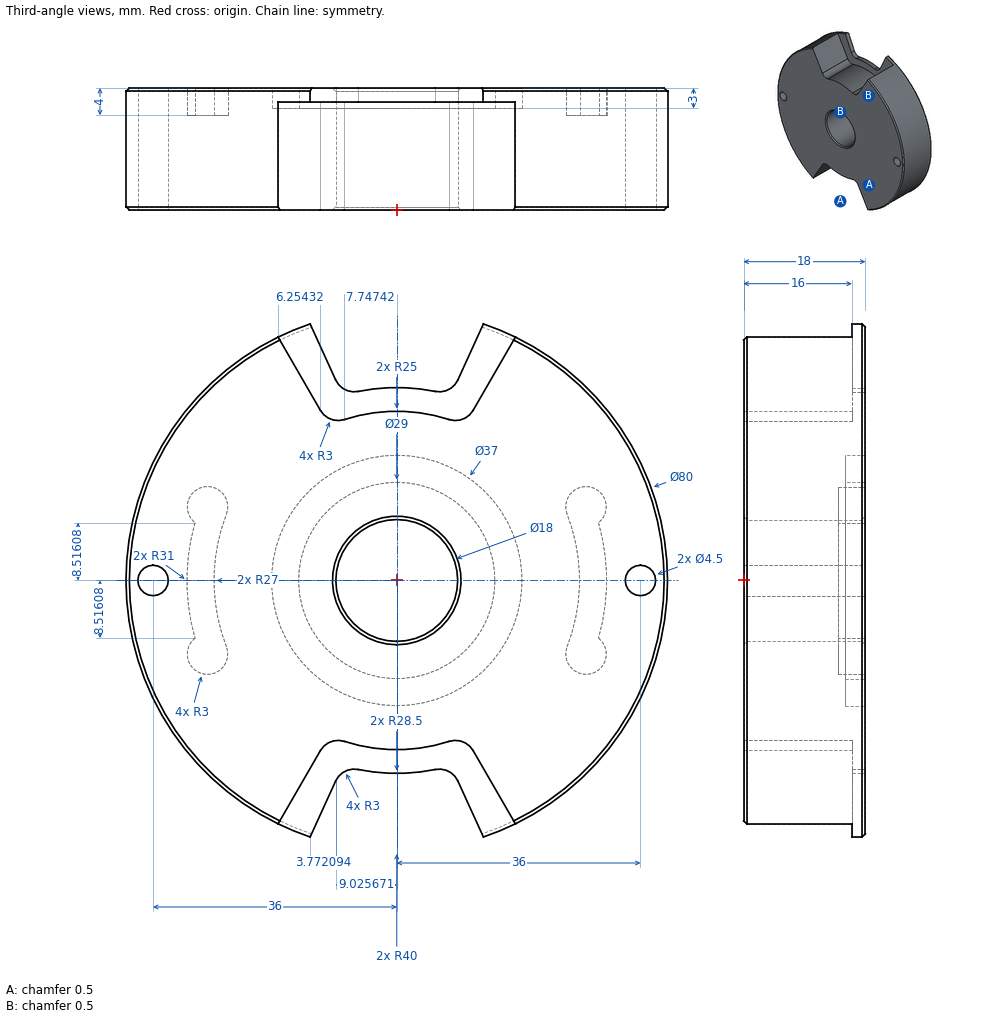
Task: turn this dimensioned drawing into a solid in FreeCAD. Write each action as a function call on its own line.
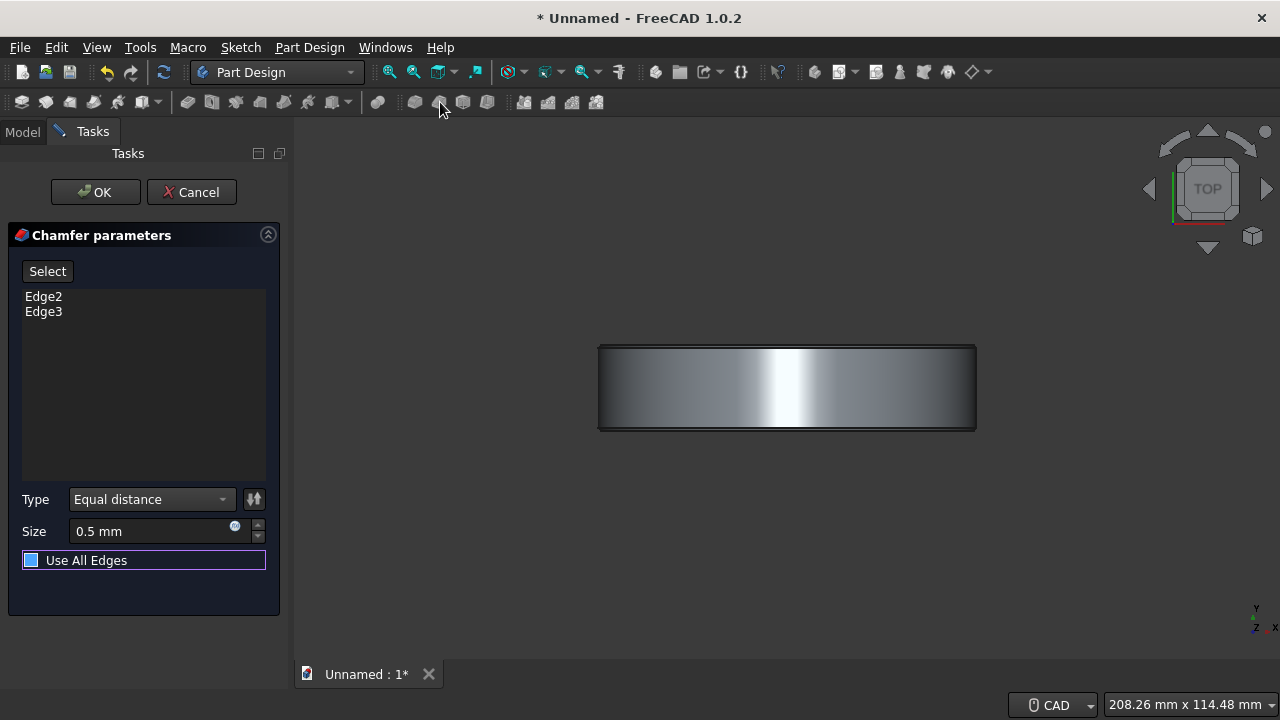
click(96, 192)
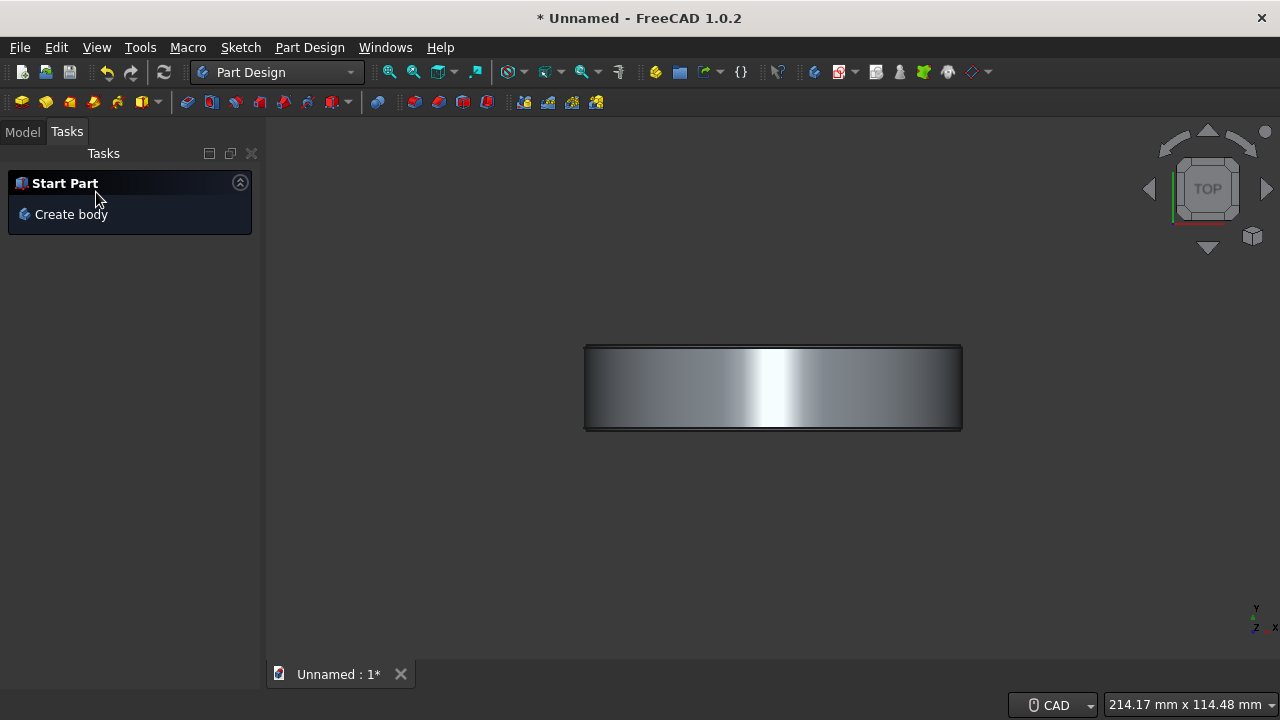
click(390, 72)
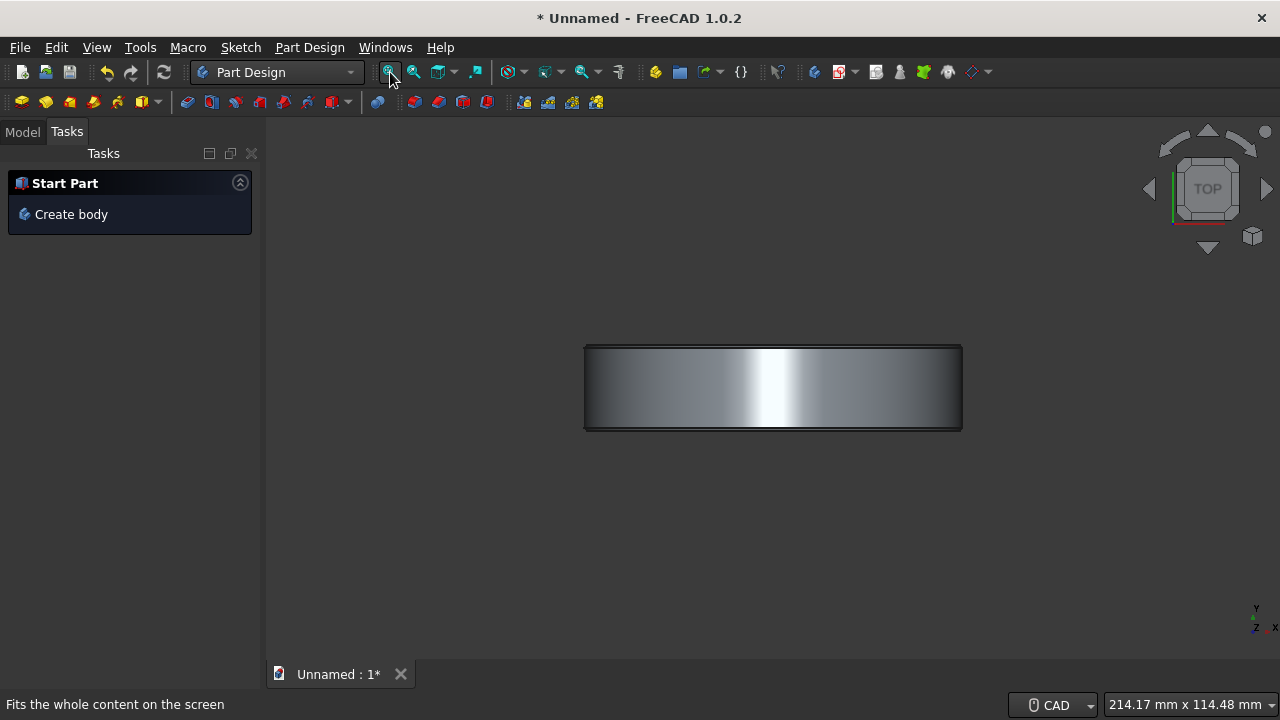
key(4)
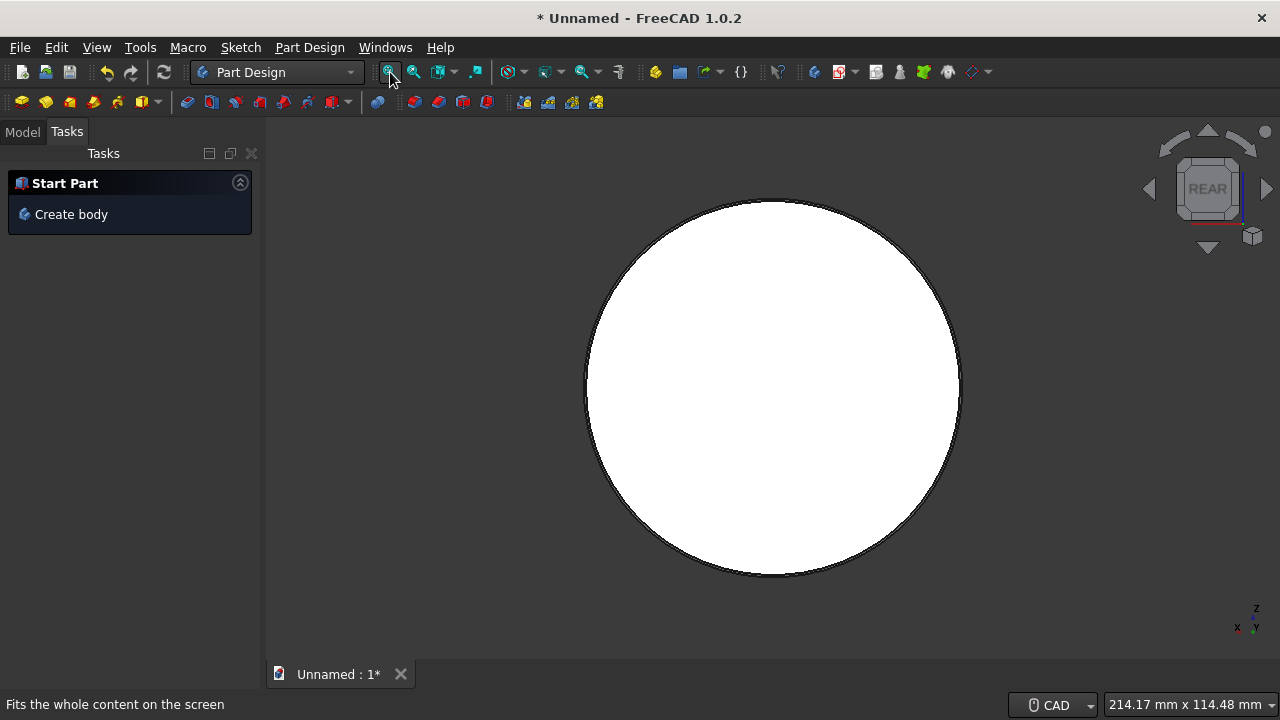
click(773, 387)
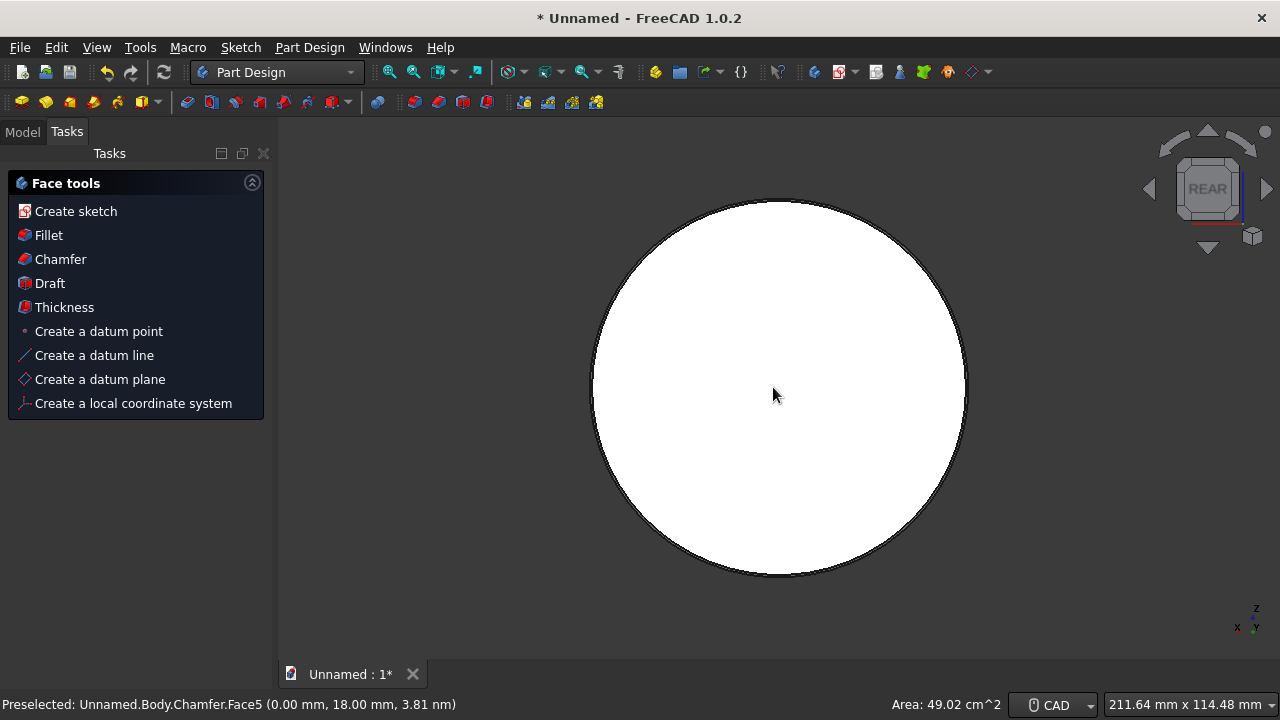
click(840, 72)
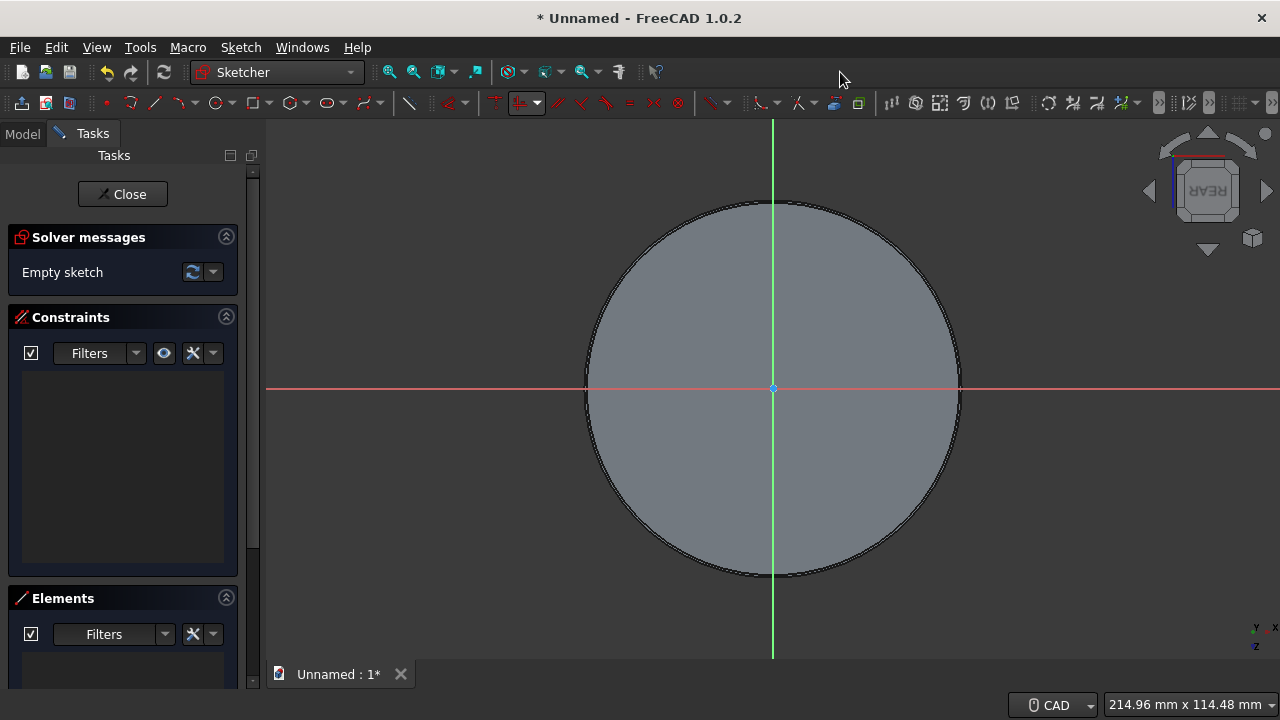
scroll(912, 389, up, 2)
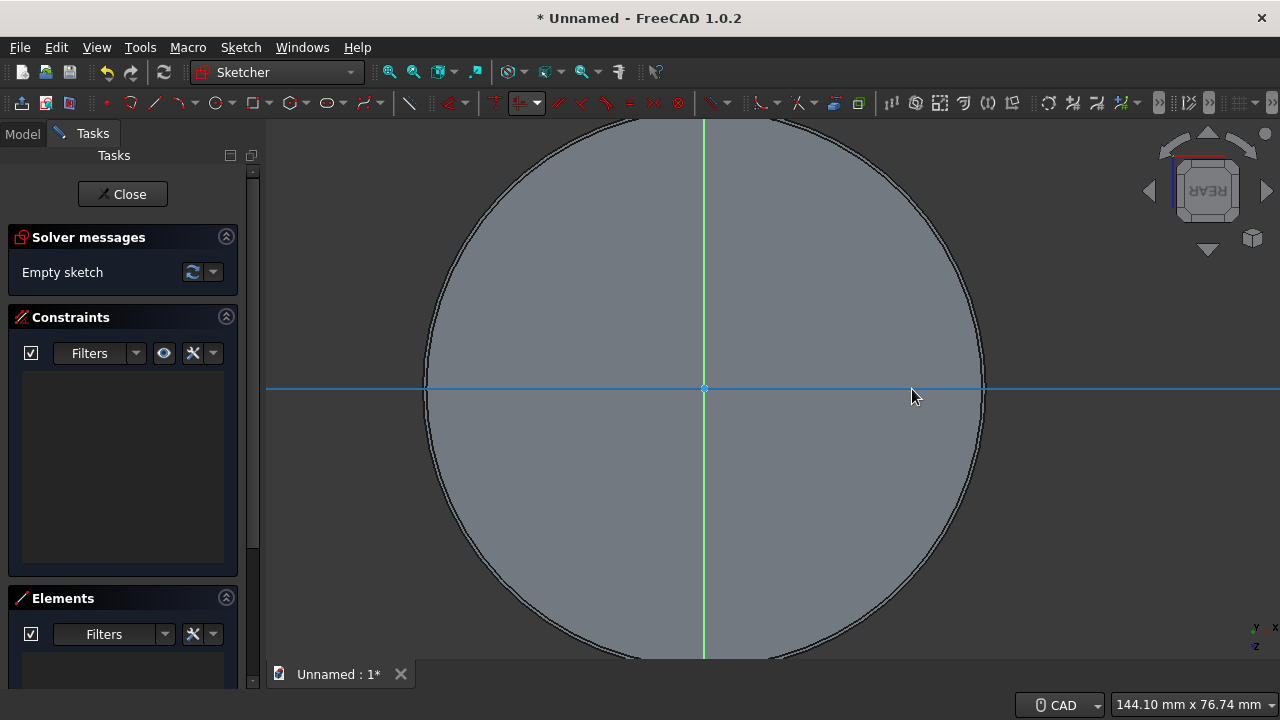
click(216, 104)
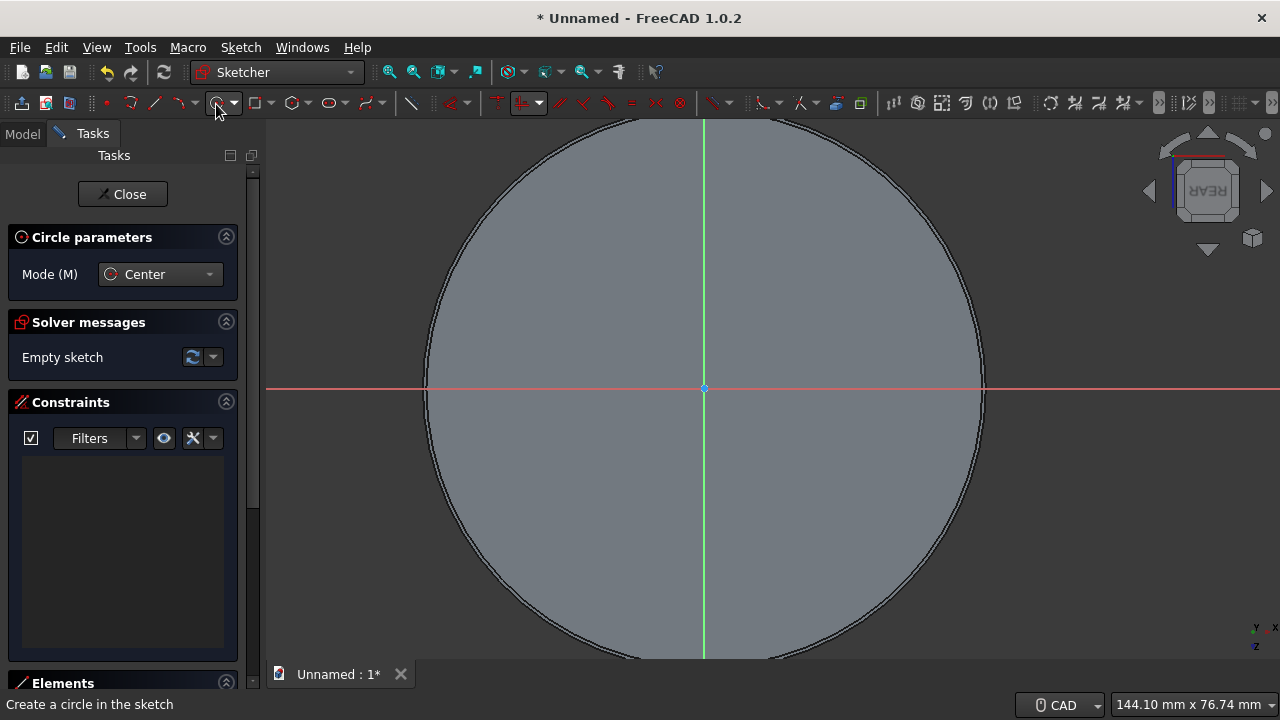
scroll(958, 389, up, 2)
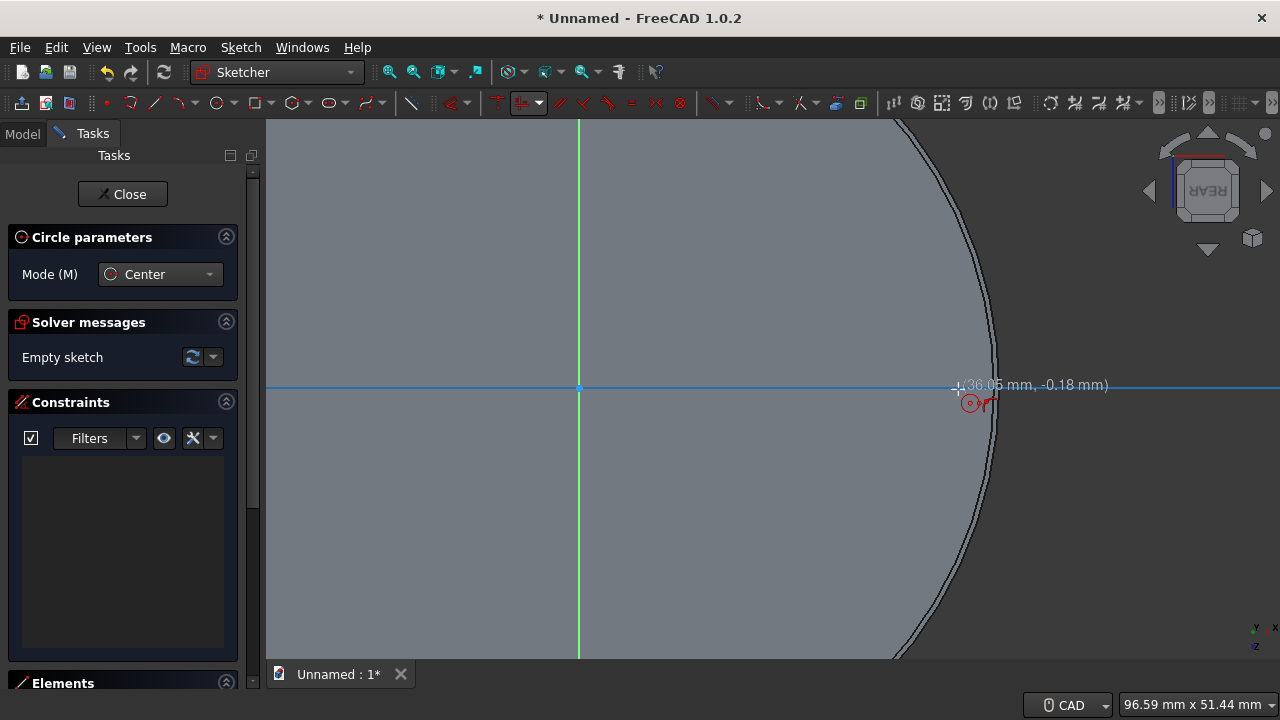
click(957, 388)
click(974, 372)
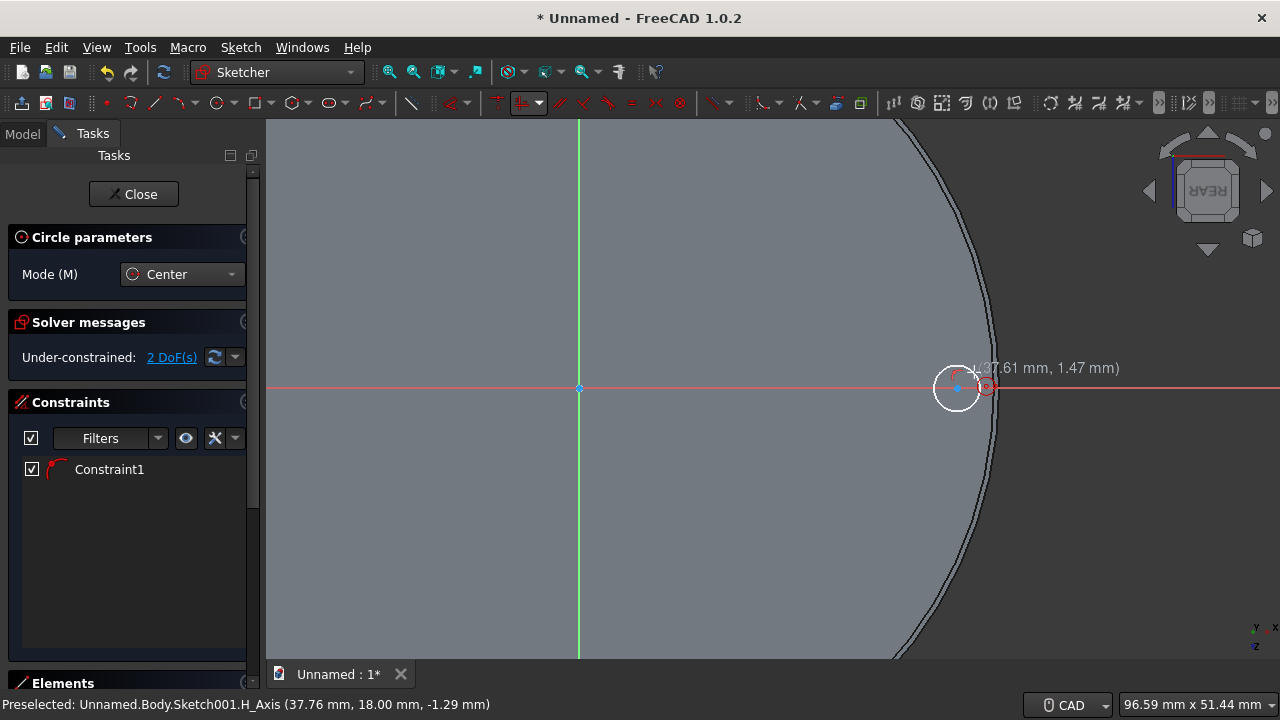
scroll(959, 390, down, 2)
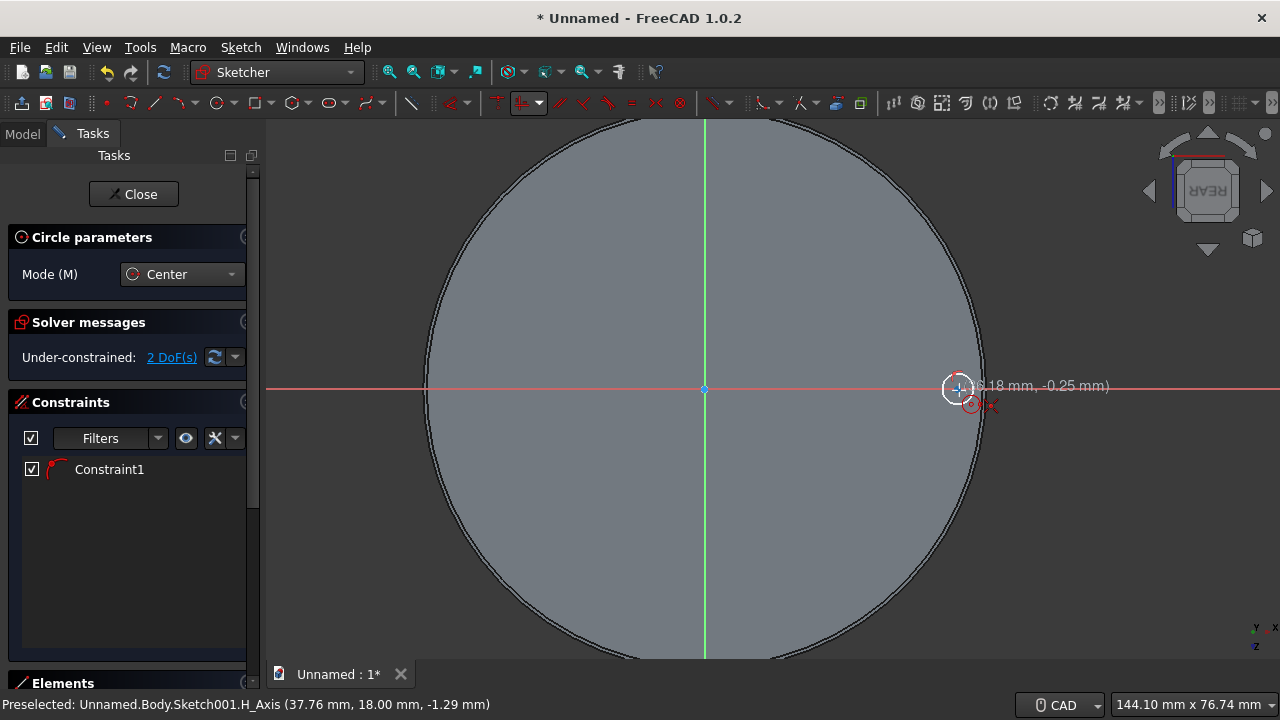
scroll(451, 389, up, 2)